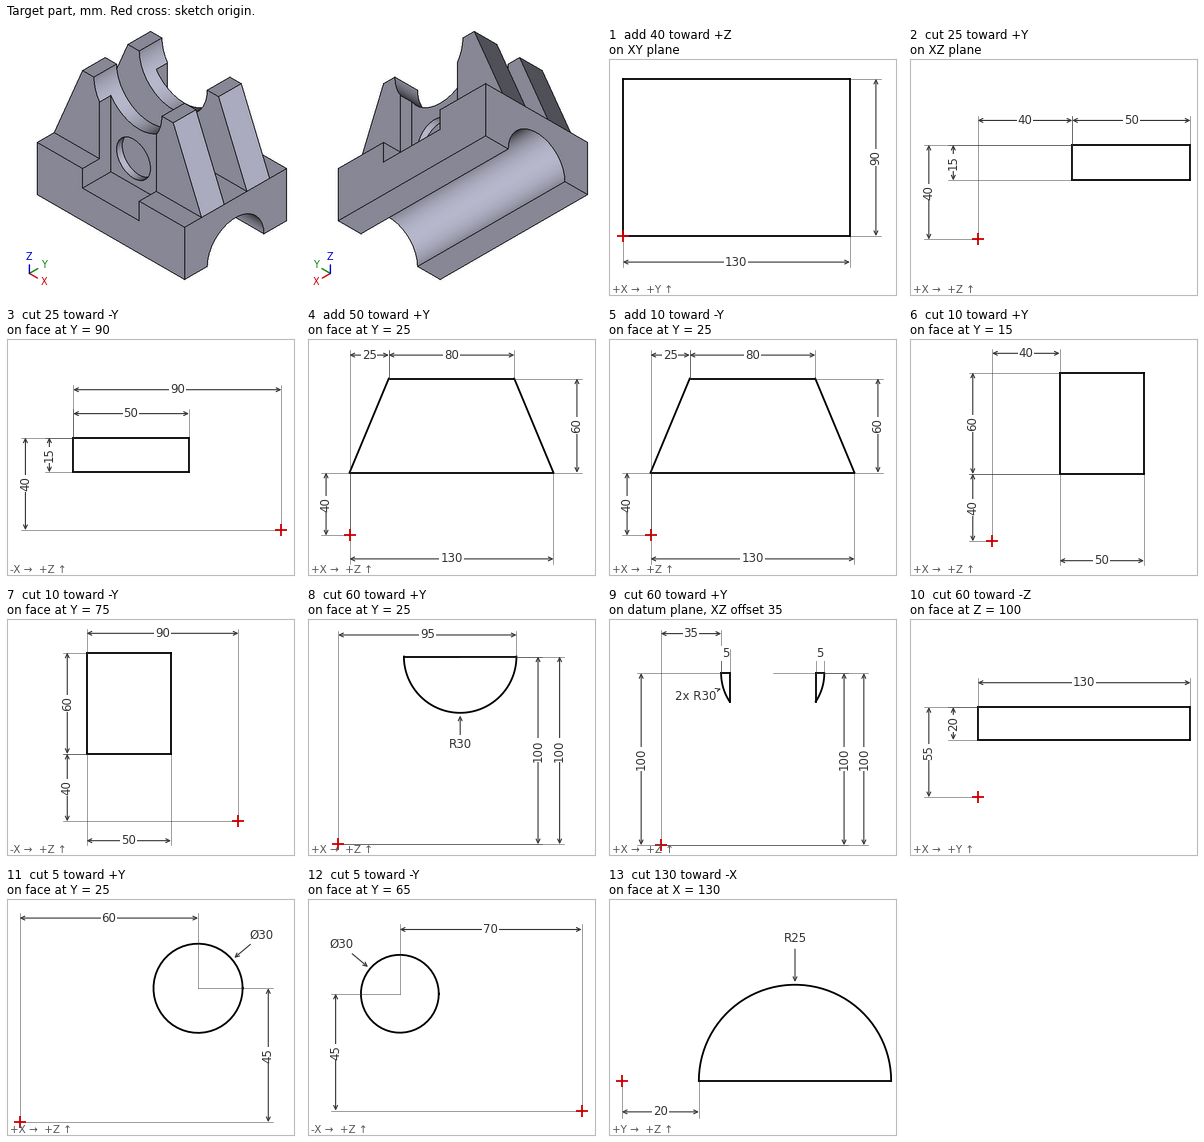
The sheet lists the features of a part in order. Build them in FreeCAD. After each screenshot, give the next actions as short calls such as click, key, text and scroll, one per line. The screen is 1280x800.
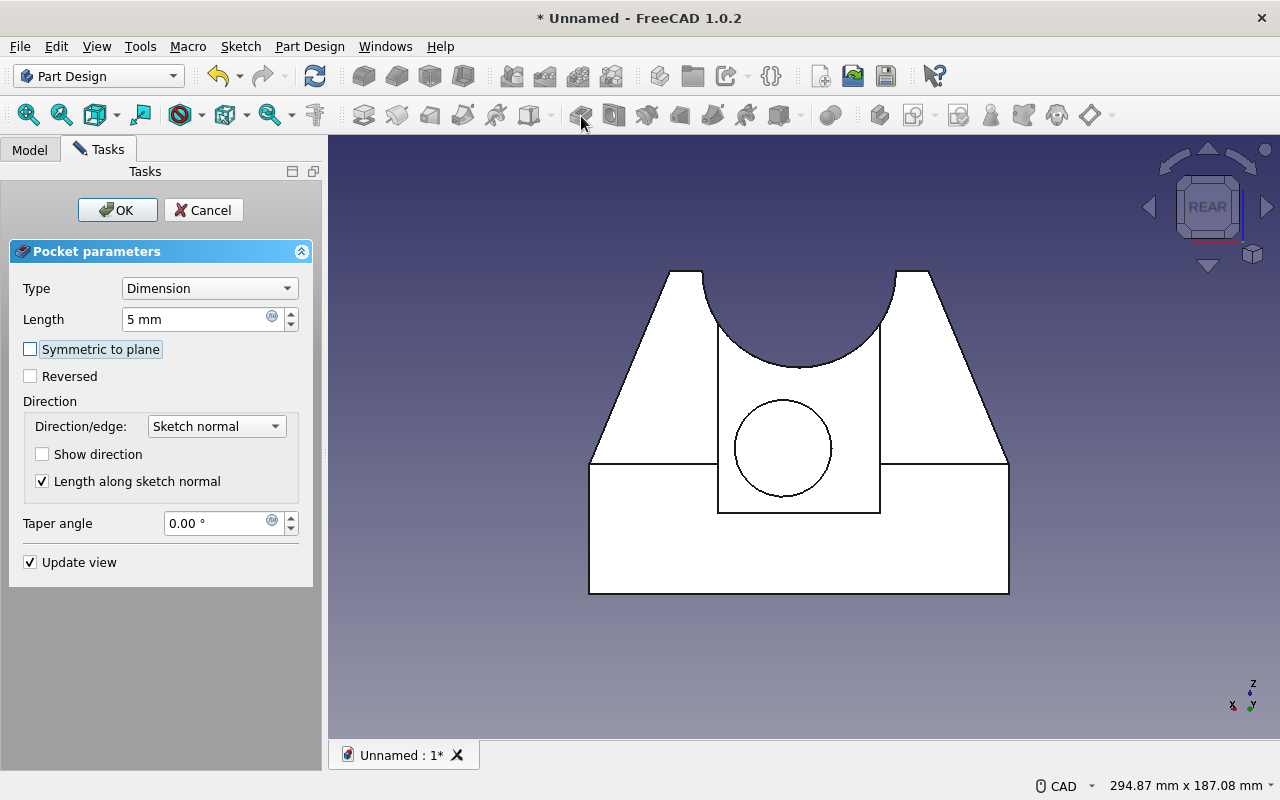
click(118, 210)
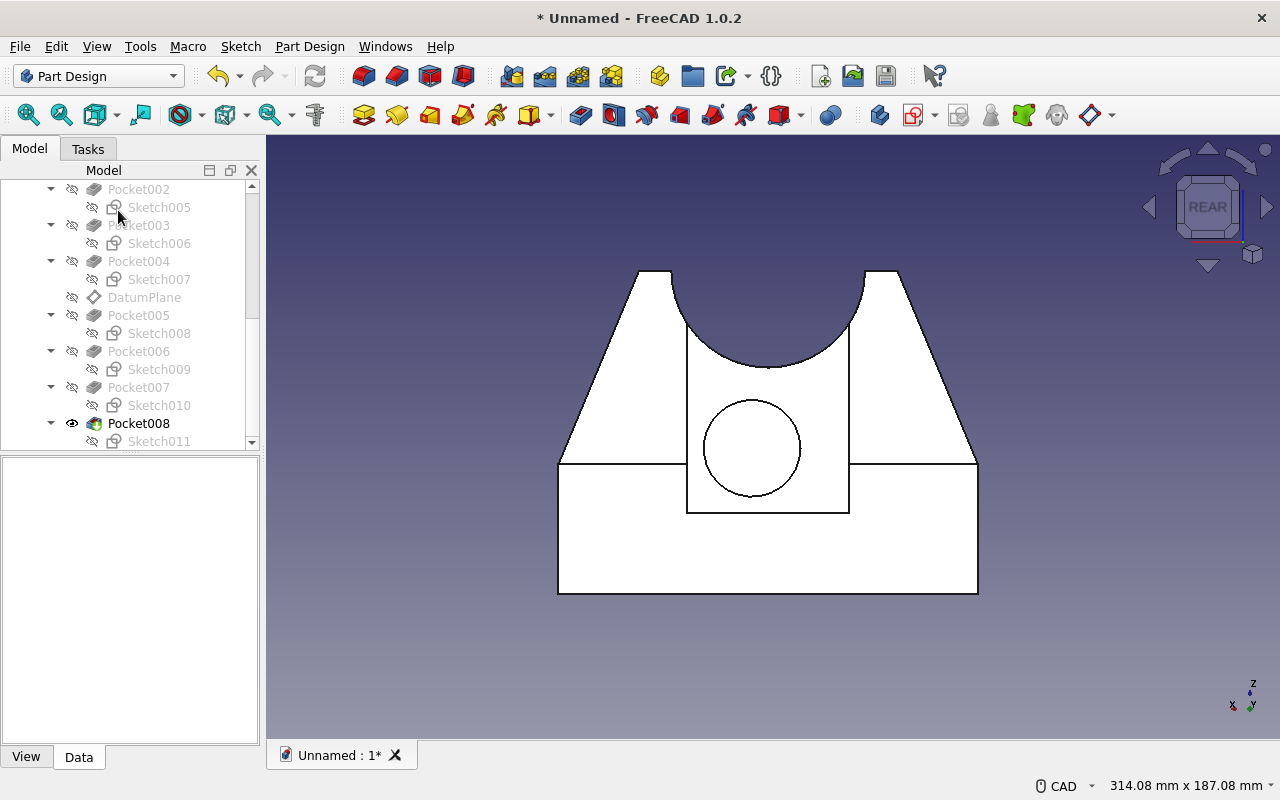
key(0)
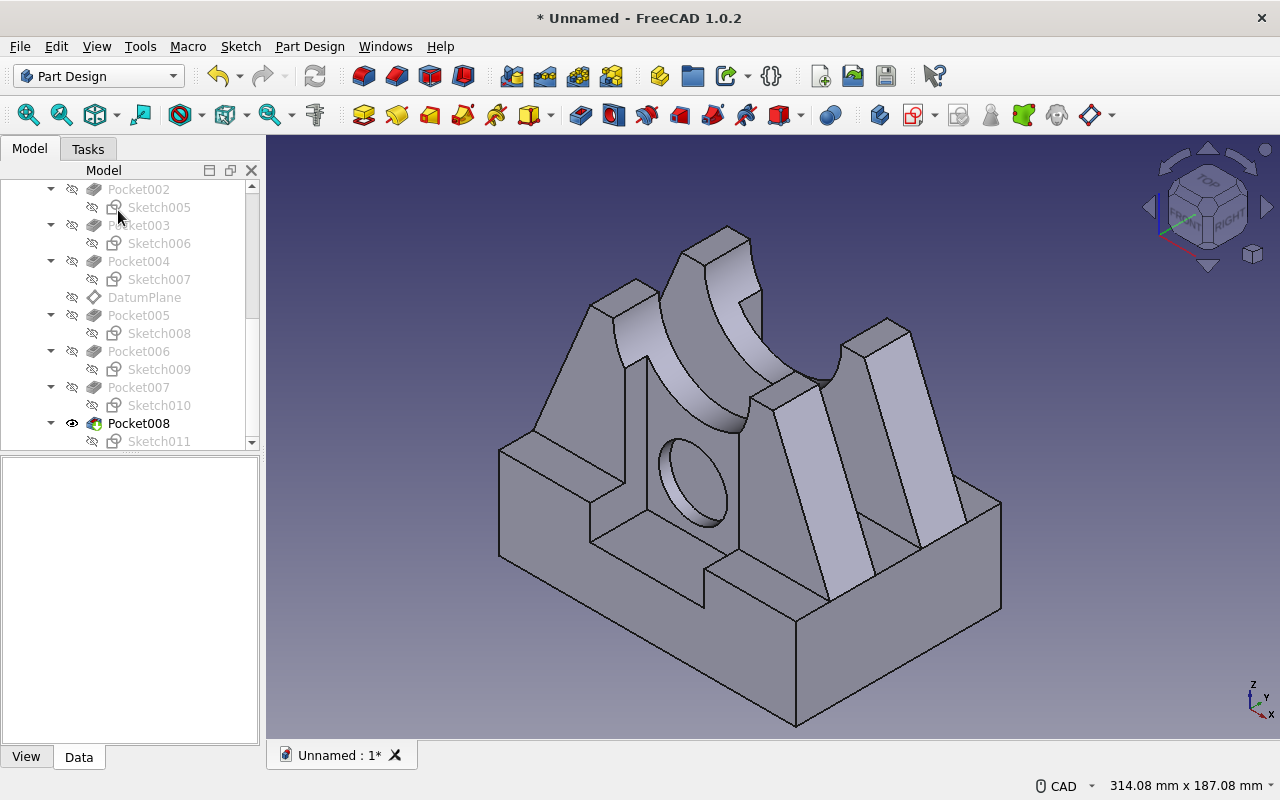
click(928, 597)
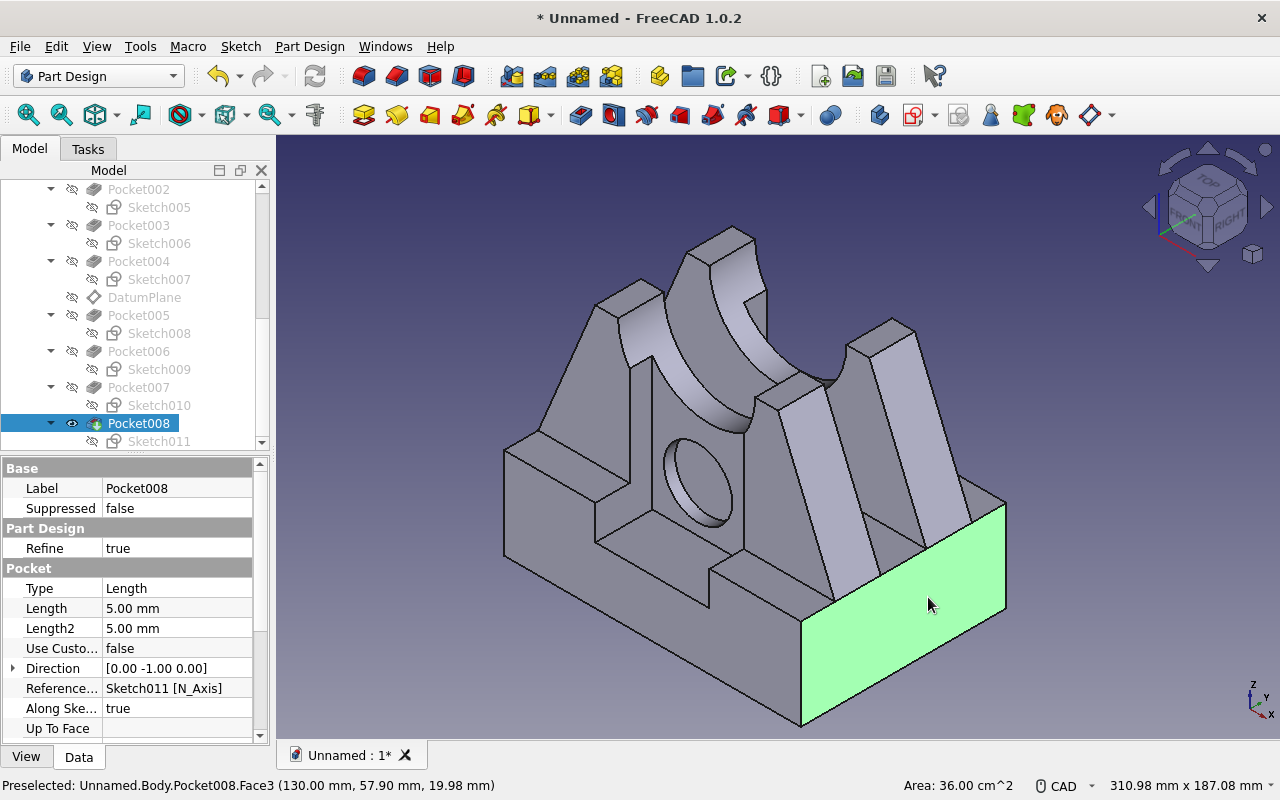
click(912, 116)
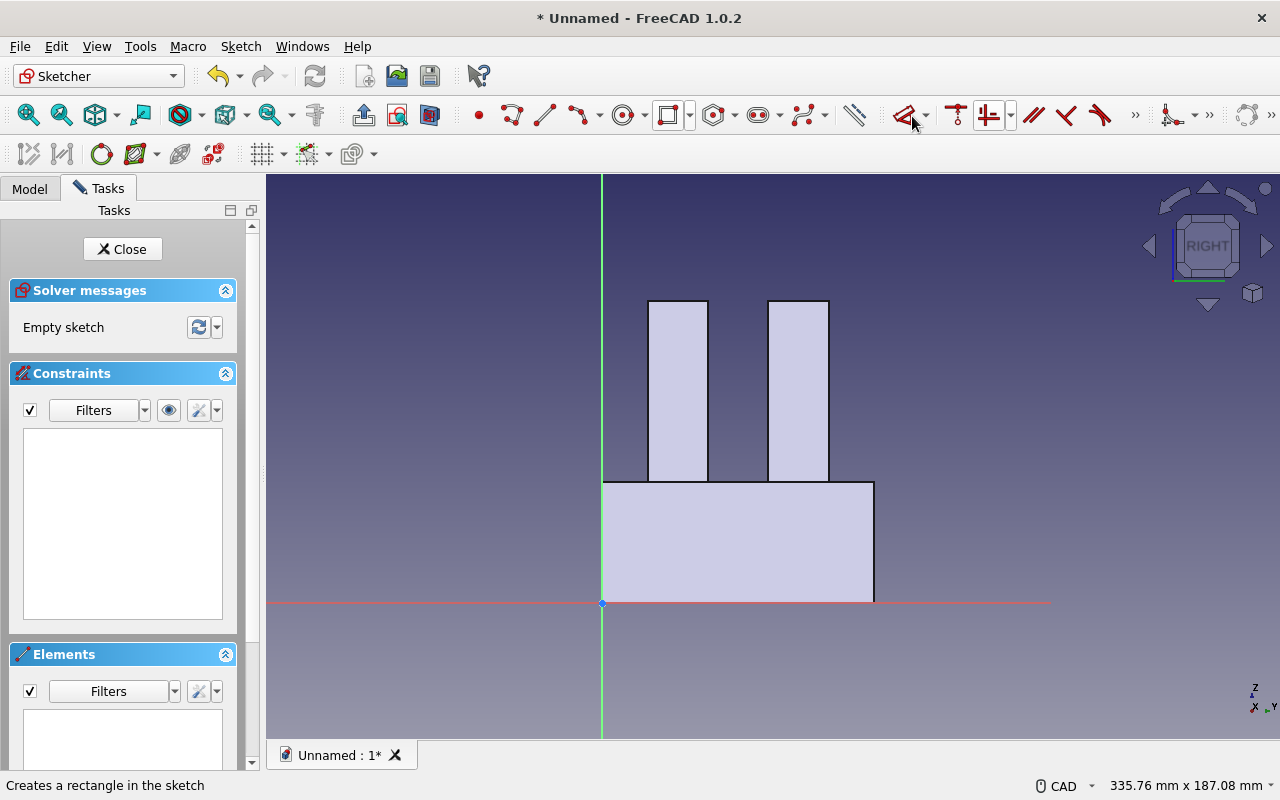
scroll(710, 629, up, 5)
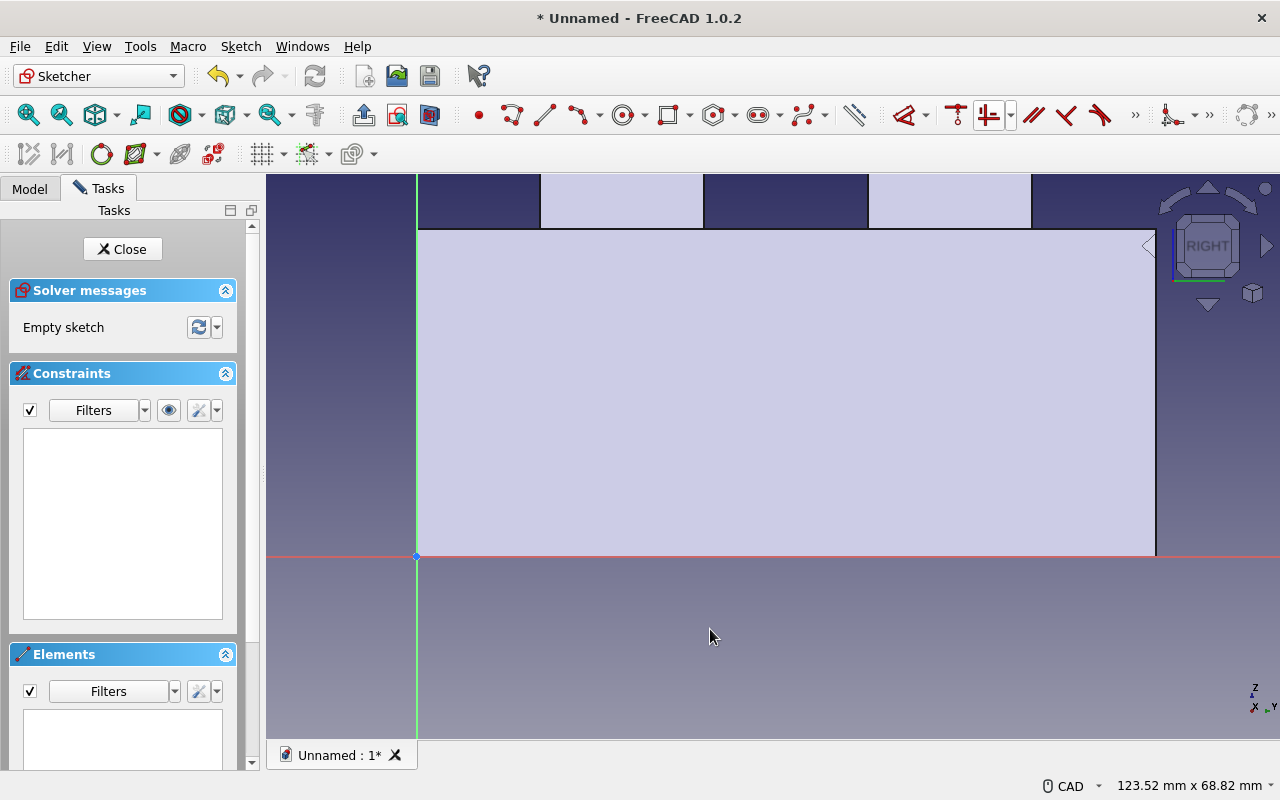
key(g)
key(l)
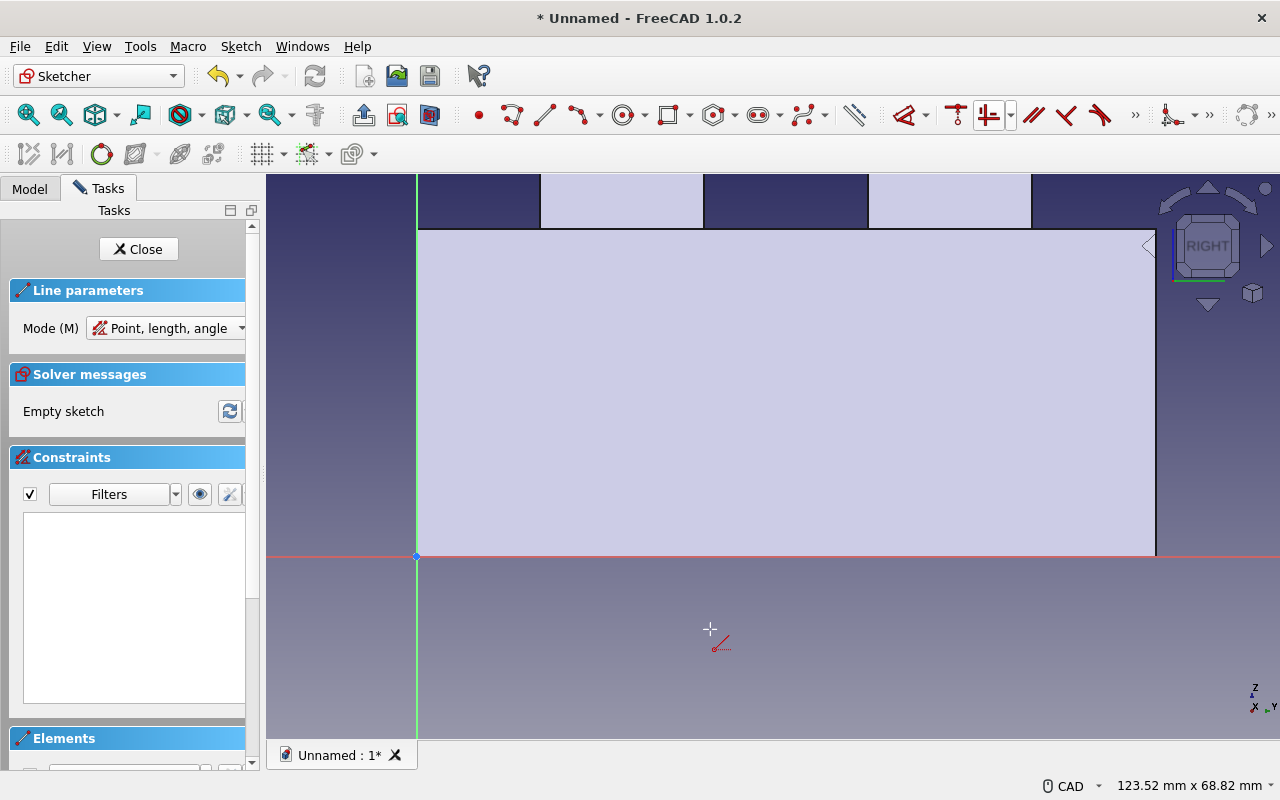
click(581, 557)
click(991, 548)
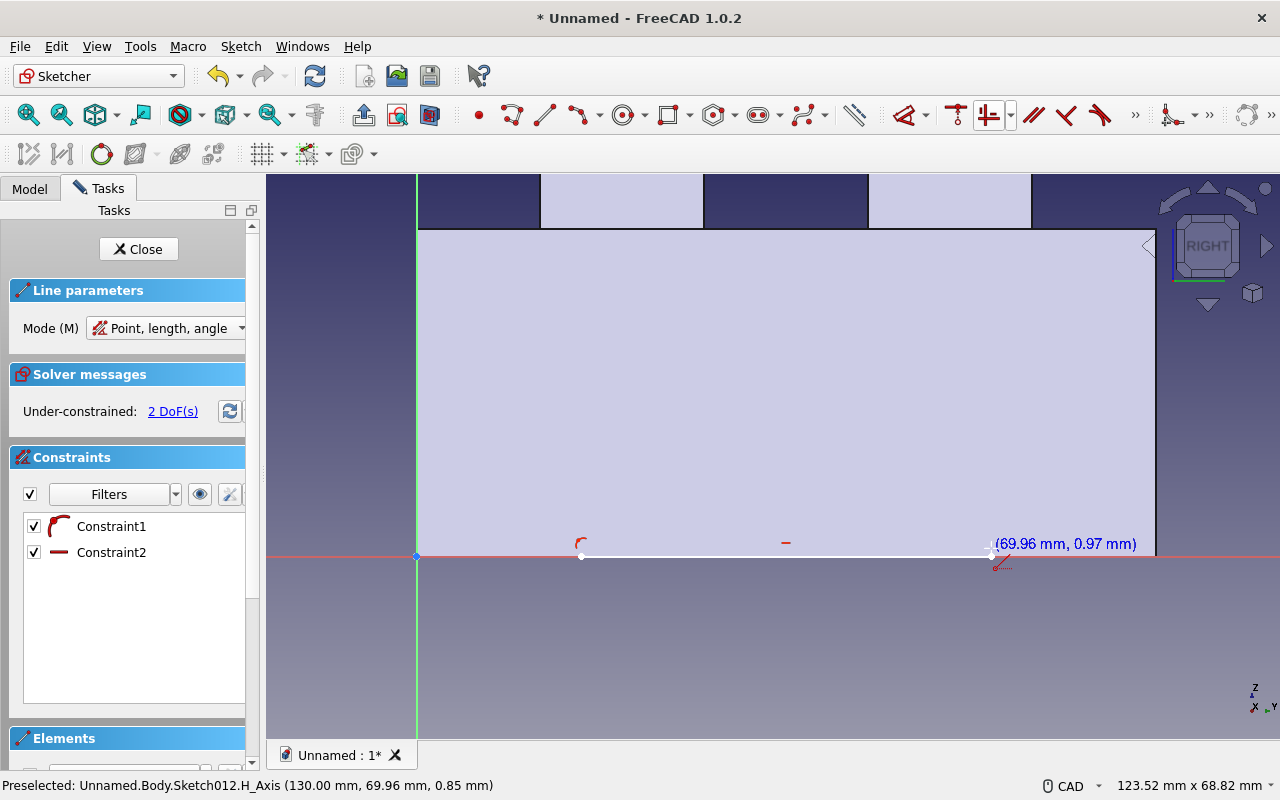
key(g)
key(3)
key(a)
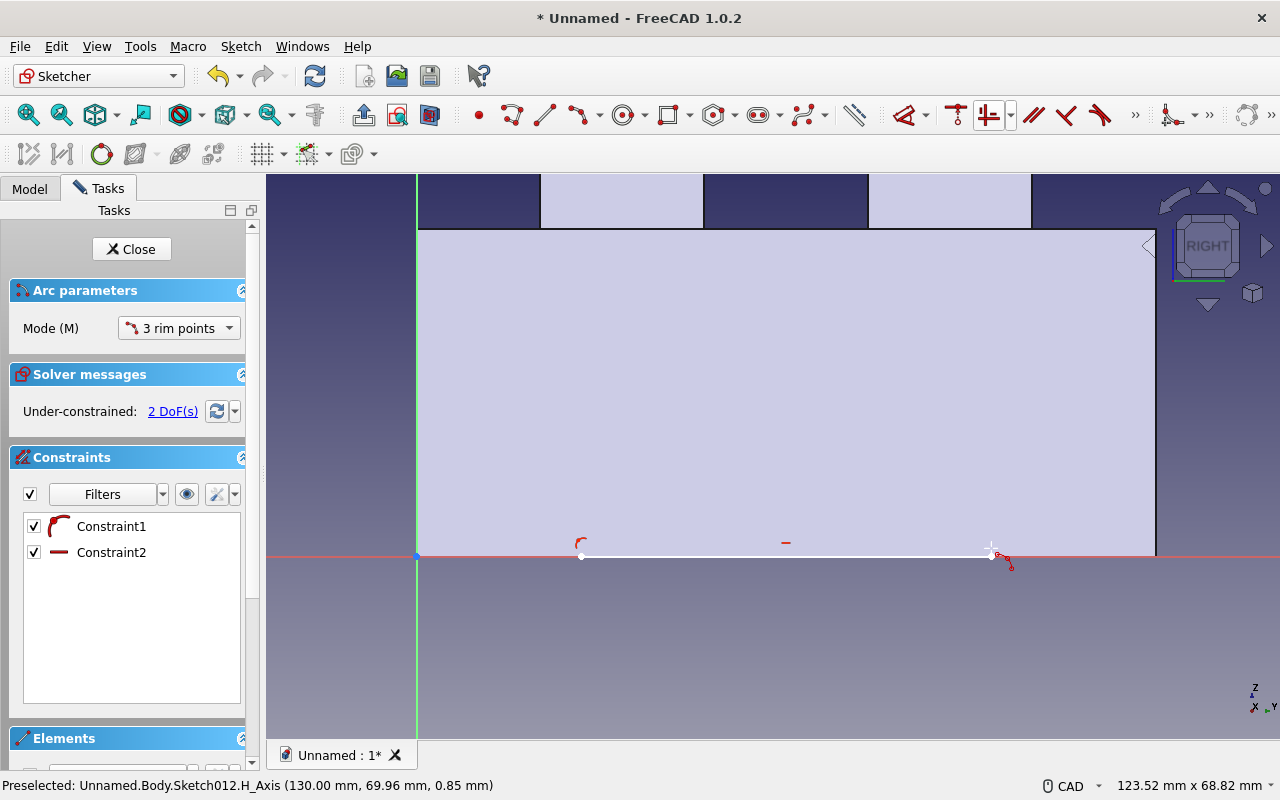
click(991, 557)
click(581, 557)
click(786, 352)
key(Escape)